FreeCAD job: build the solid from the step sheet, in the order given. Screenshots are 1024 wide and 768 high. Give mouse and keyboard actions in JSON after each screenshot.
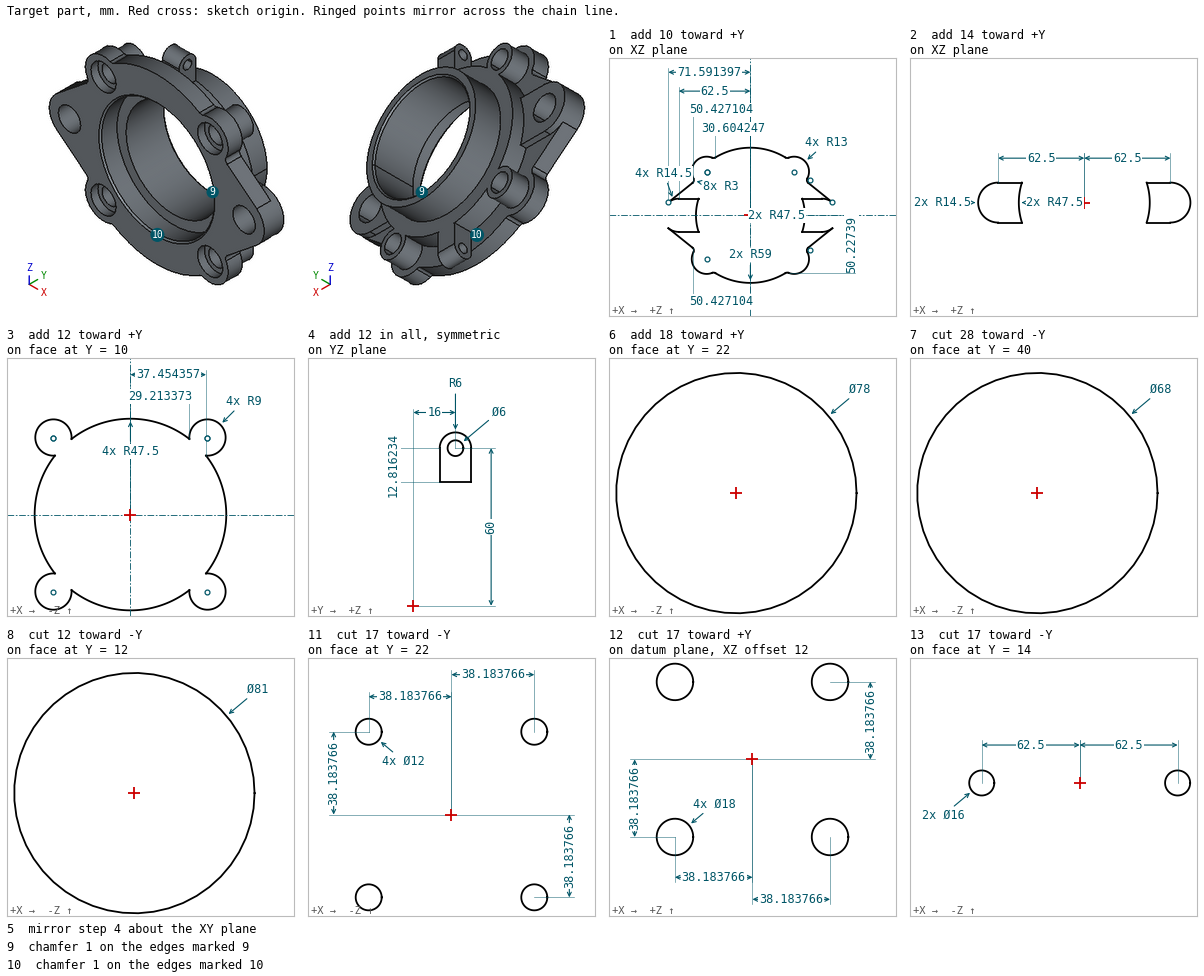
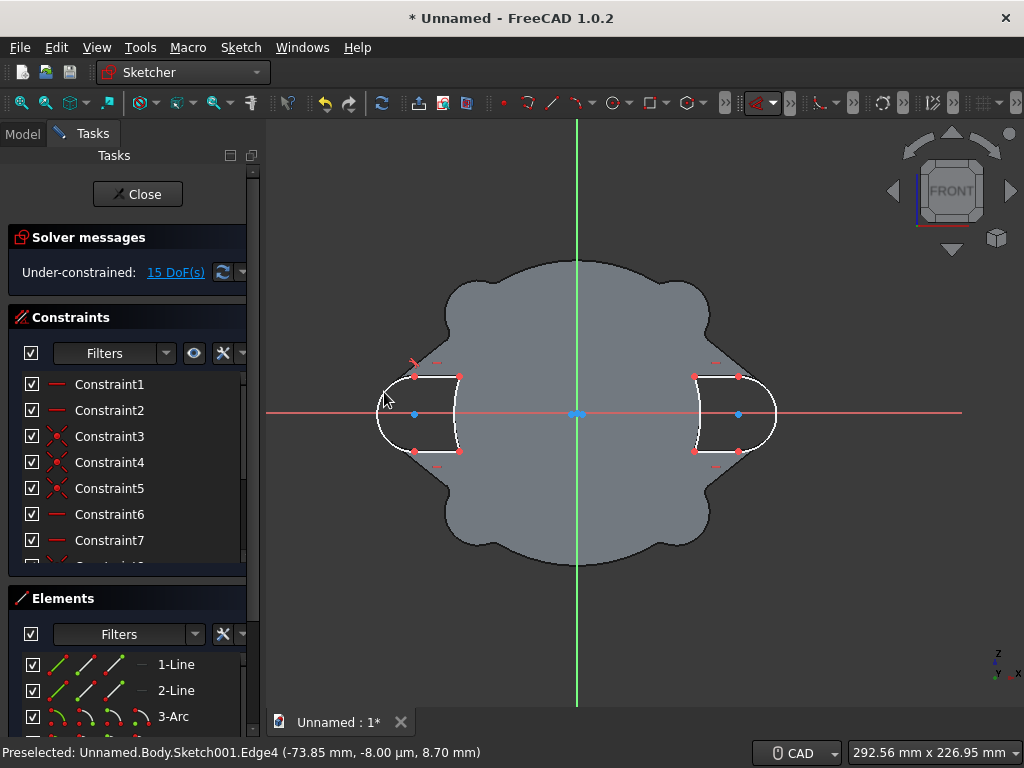
{"action": "left_click", "coordinate": [446, 452]}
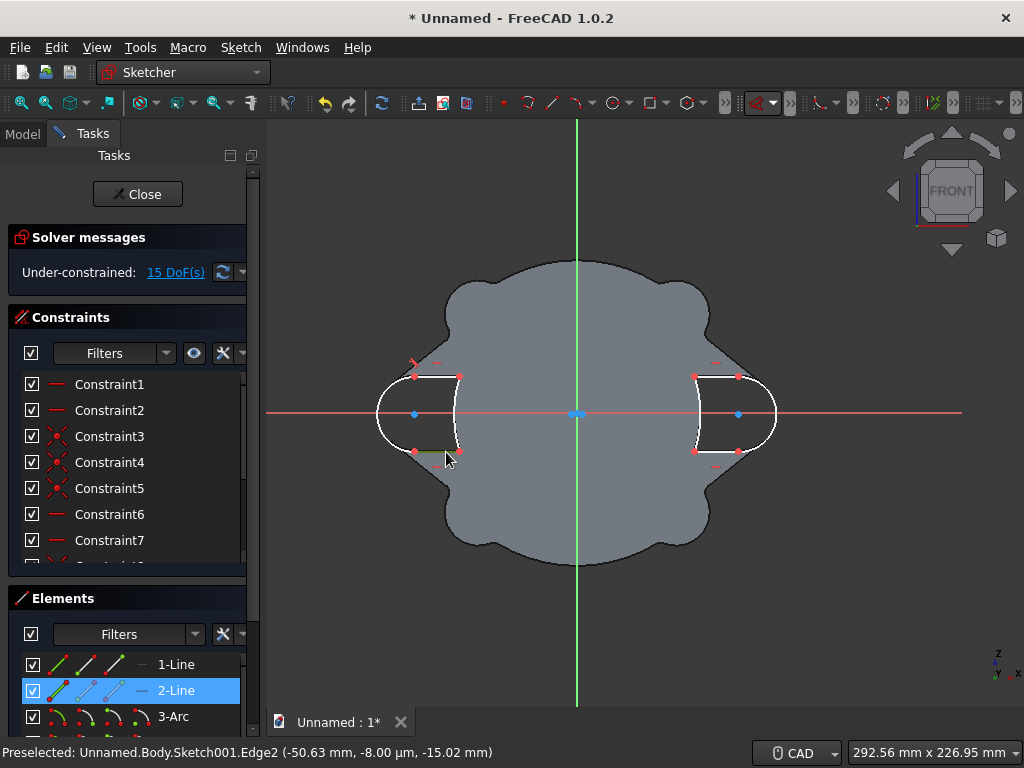
{"action": "left_click", "coordinate": [384, 392]}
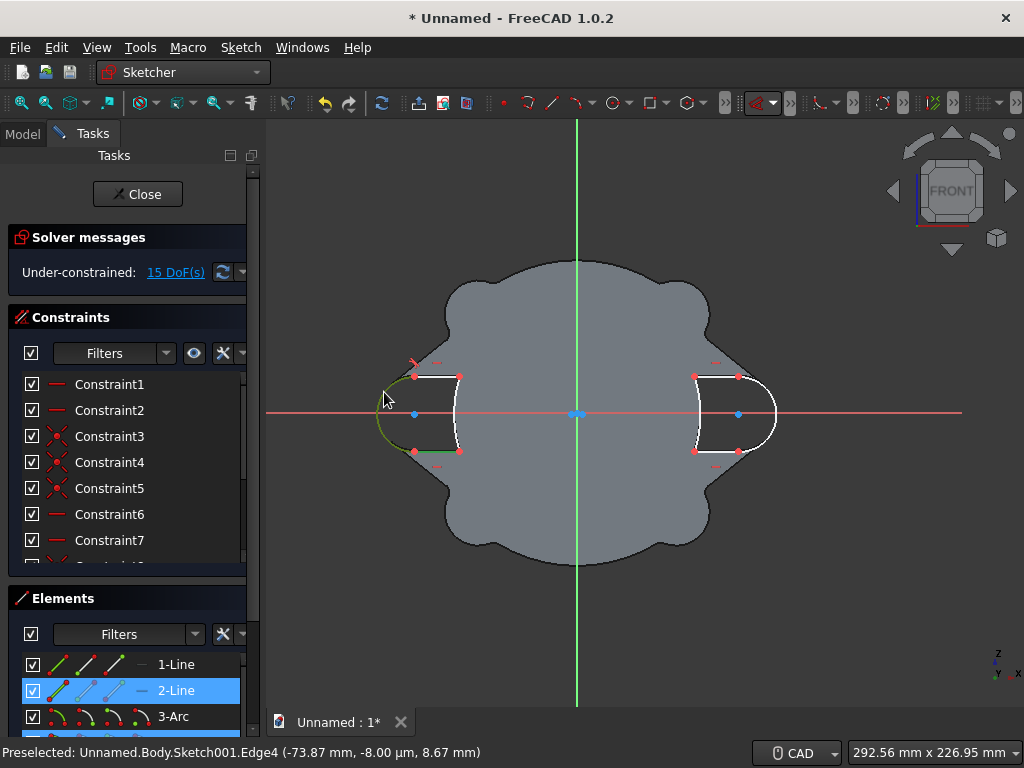
{"action": "key", "text": "t"}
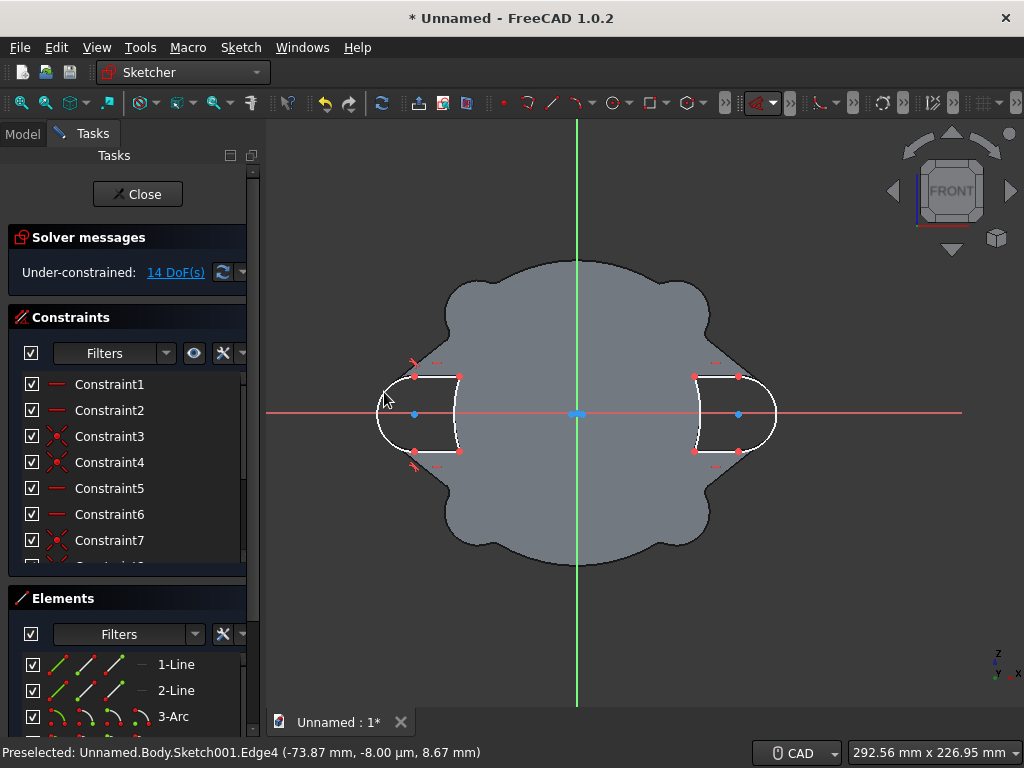
{"action": "left_click", "coordinate": [708, 377]}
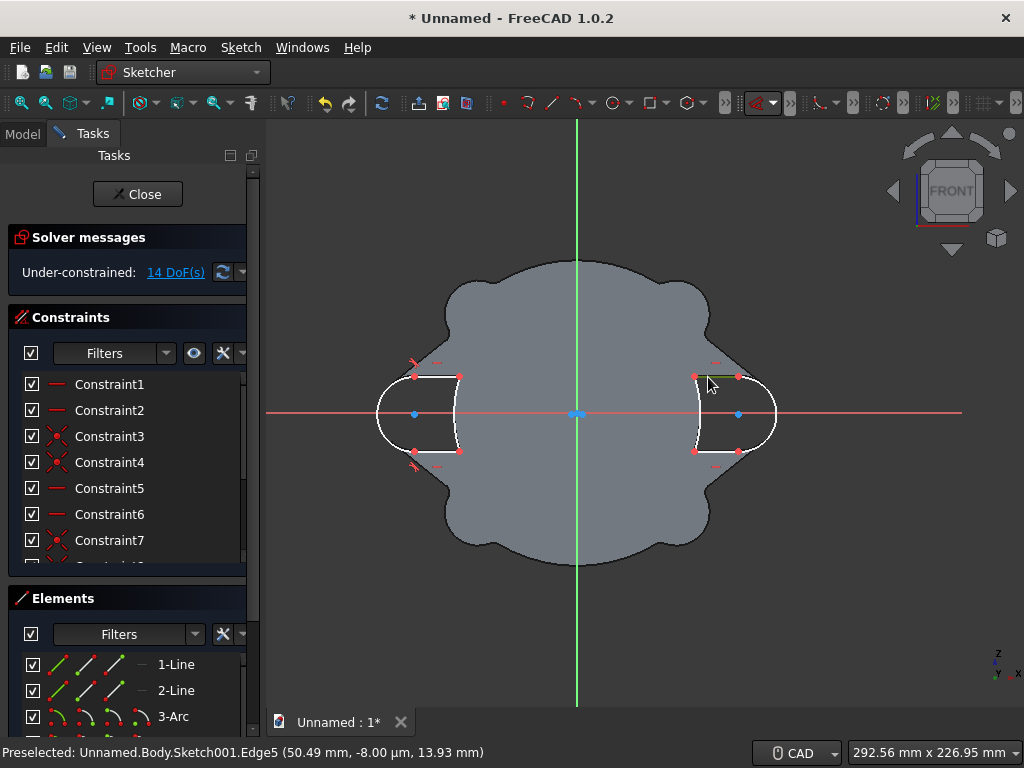
{"action": "left_click", "coordinate": [769, 437]}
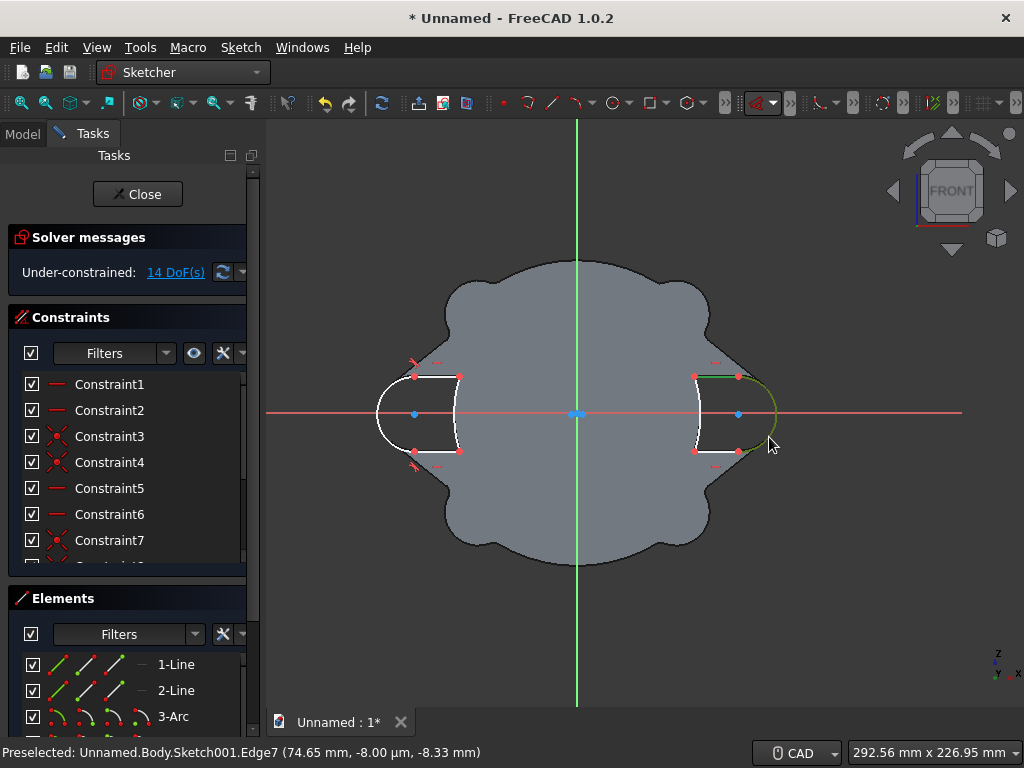
{"action": "key", "text": "t"}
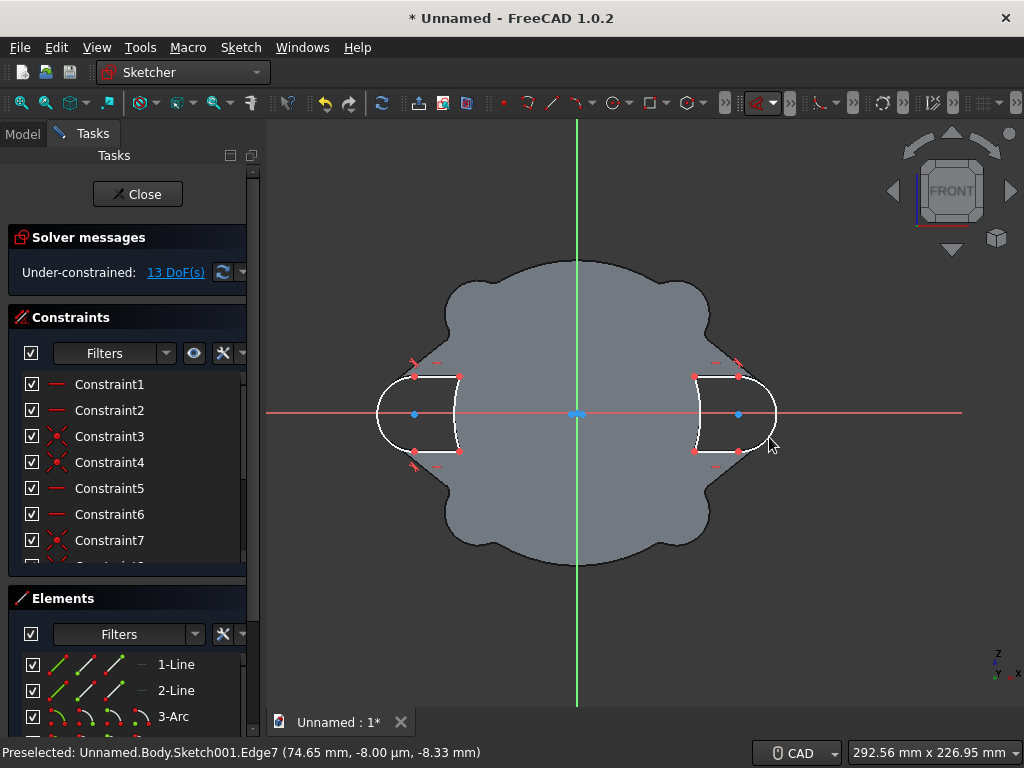
{"action": "left_click", "coordinate": [725, 452]}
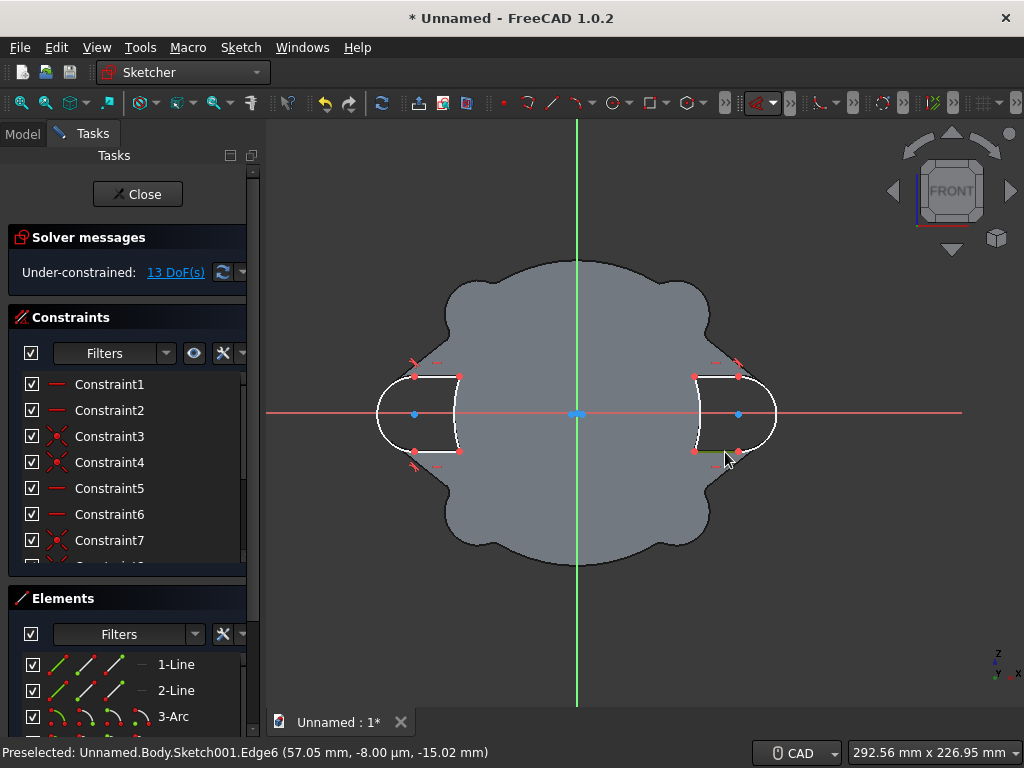
{"action": "left_click", "coordinate": [769, 437]}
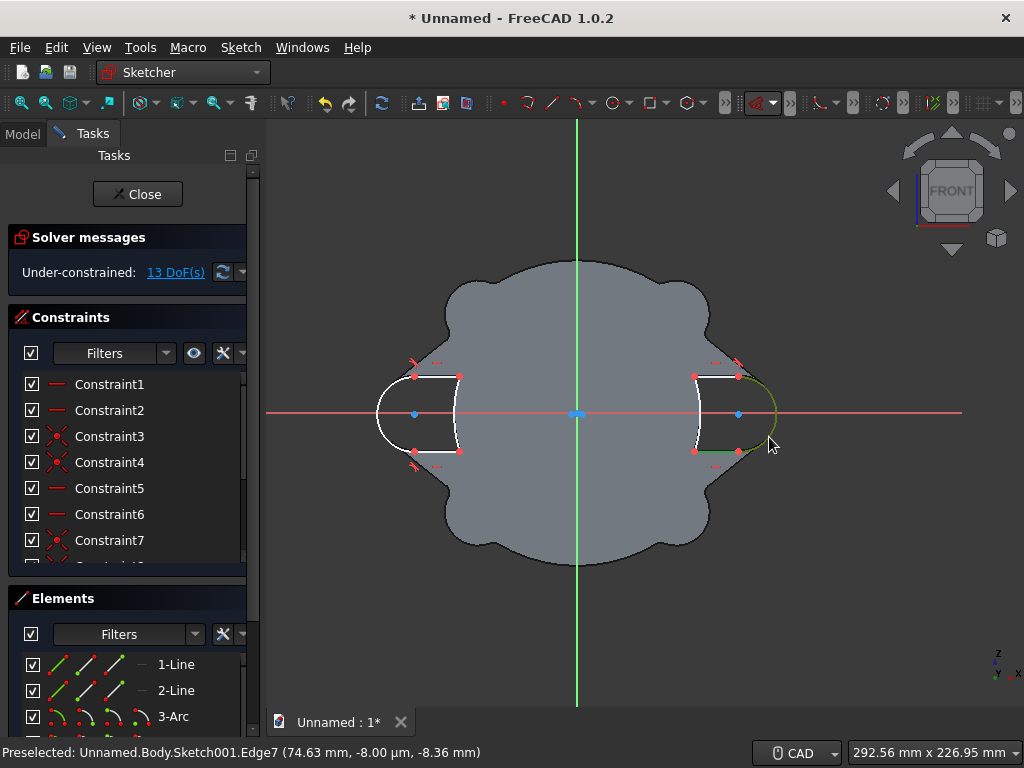
{"action": "key", "text": "t"}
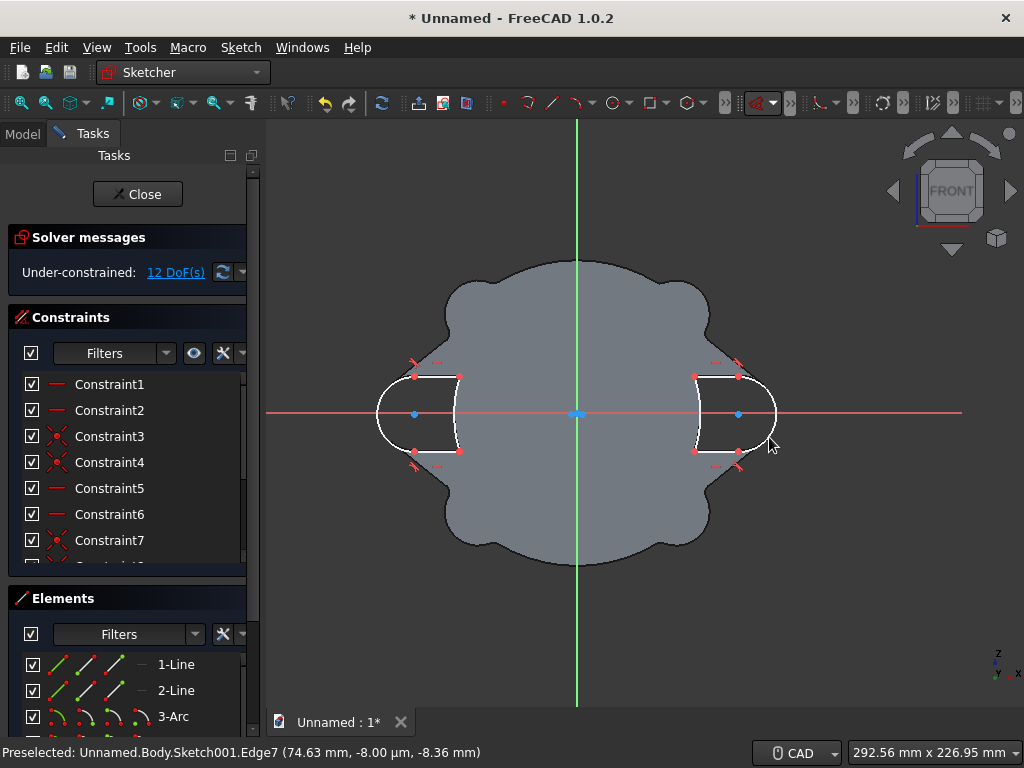
{"action": "left_click", "coordinate": [455, 399]}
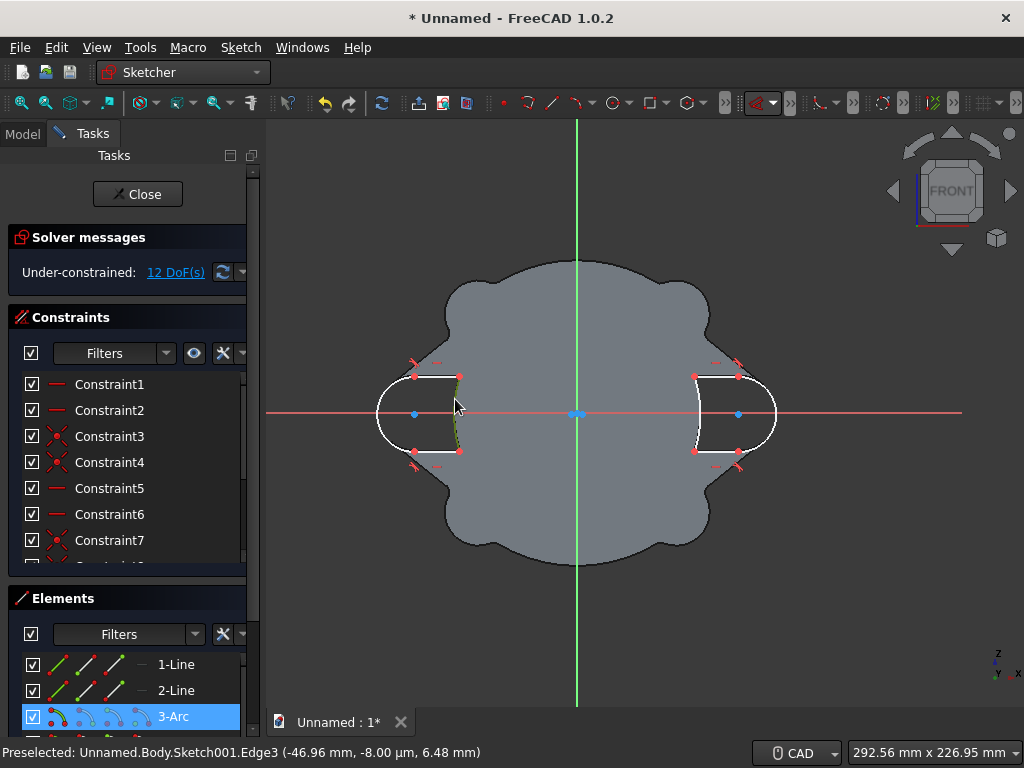
{"action": "left_click", "coordinate": [699, 430]}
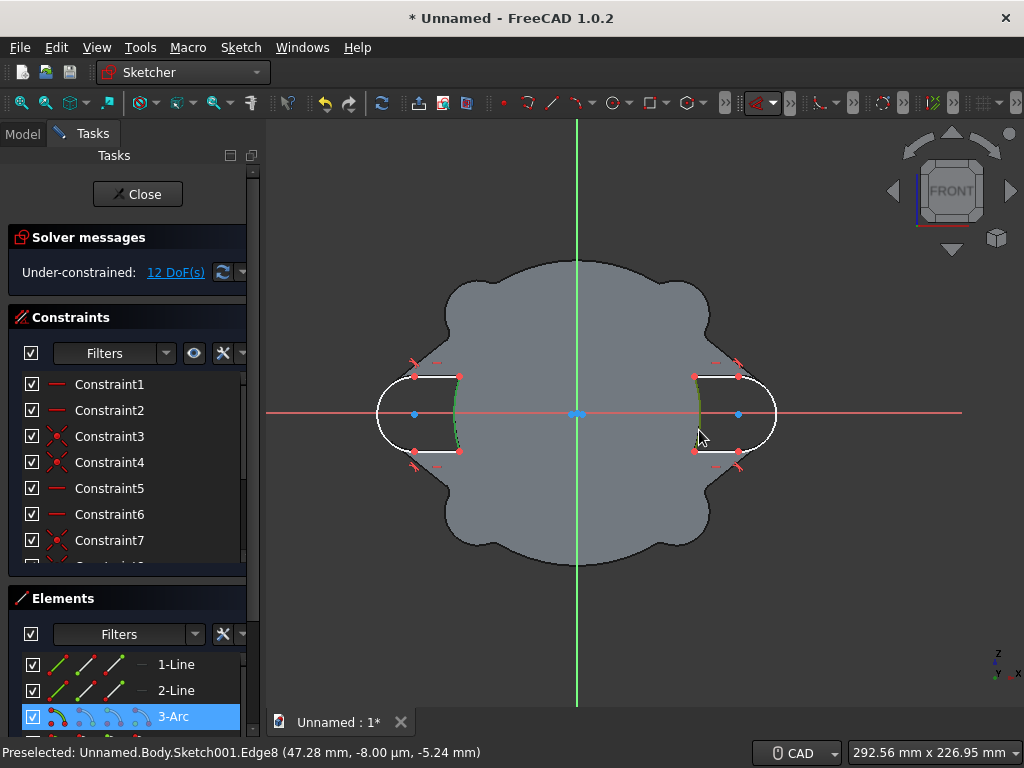
{"action": "key", "text": "c"}